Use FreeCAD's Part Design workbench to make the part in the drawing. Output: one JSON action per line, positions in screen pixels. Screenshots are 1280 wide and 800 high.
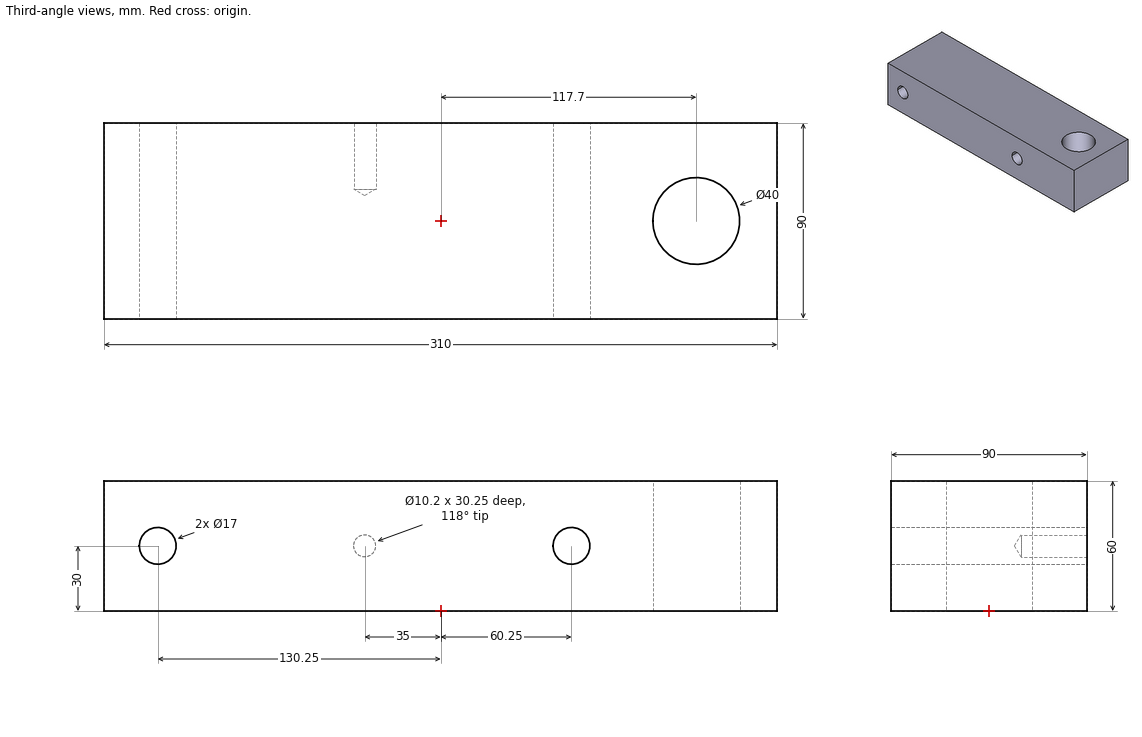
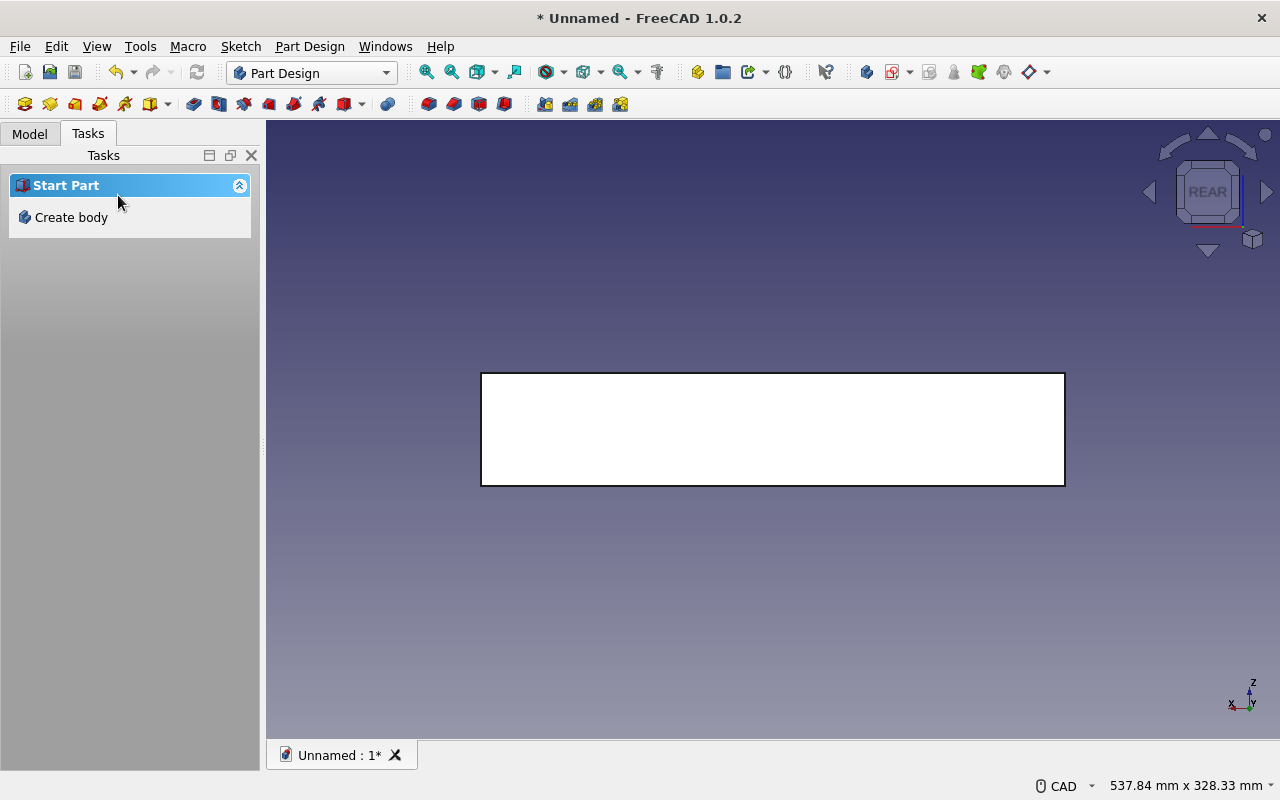
{"action": "left_click", "coordinate": [606, 429]}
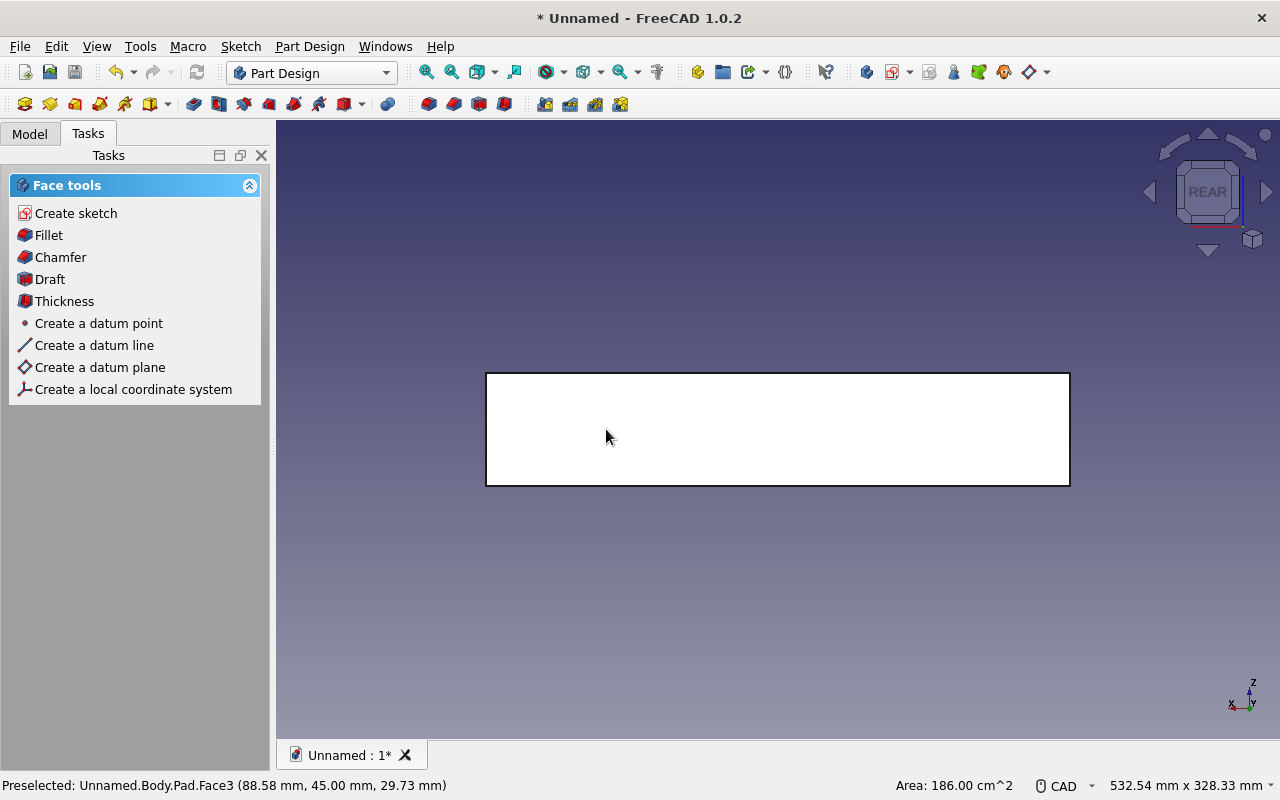
{"action": "left_click", "coordinate": [892, 72]}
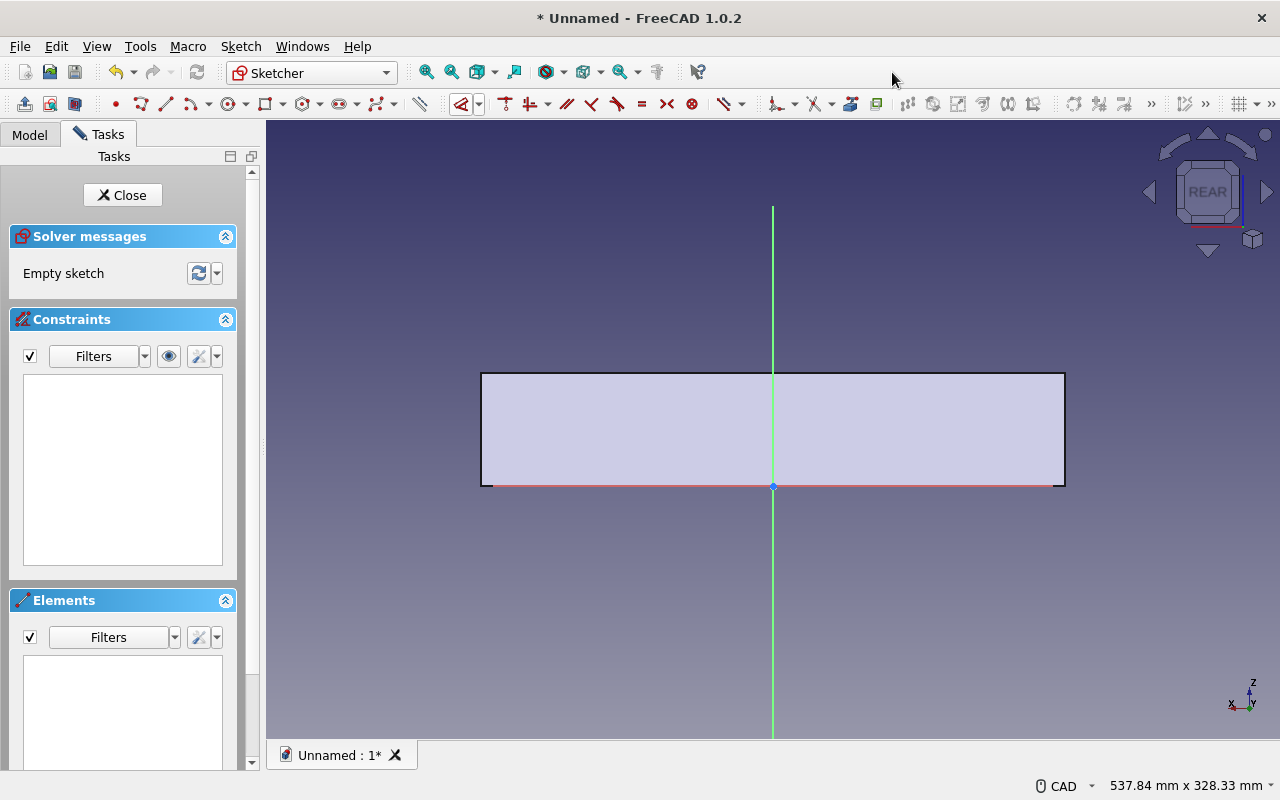
{"action": "scroll", "coordinate": [1112, 491], "scroll_direction": "up", "scroll_amount": 2}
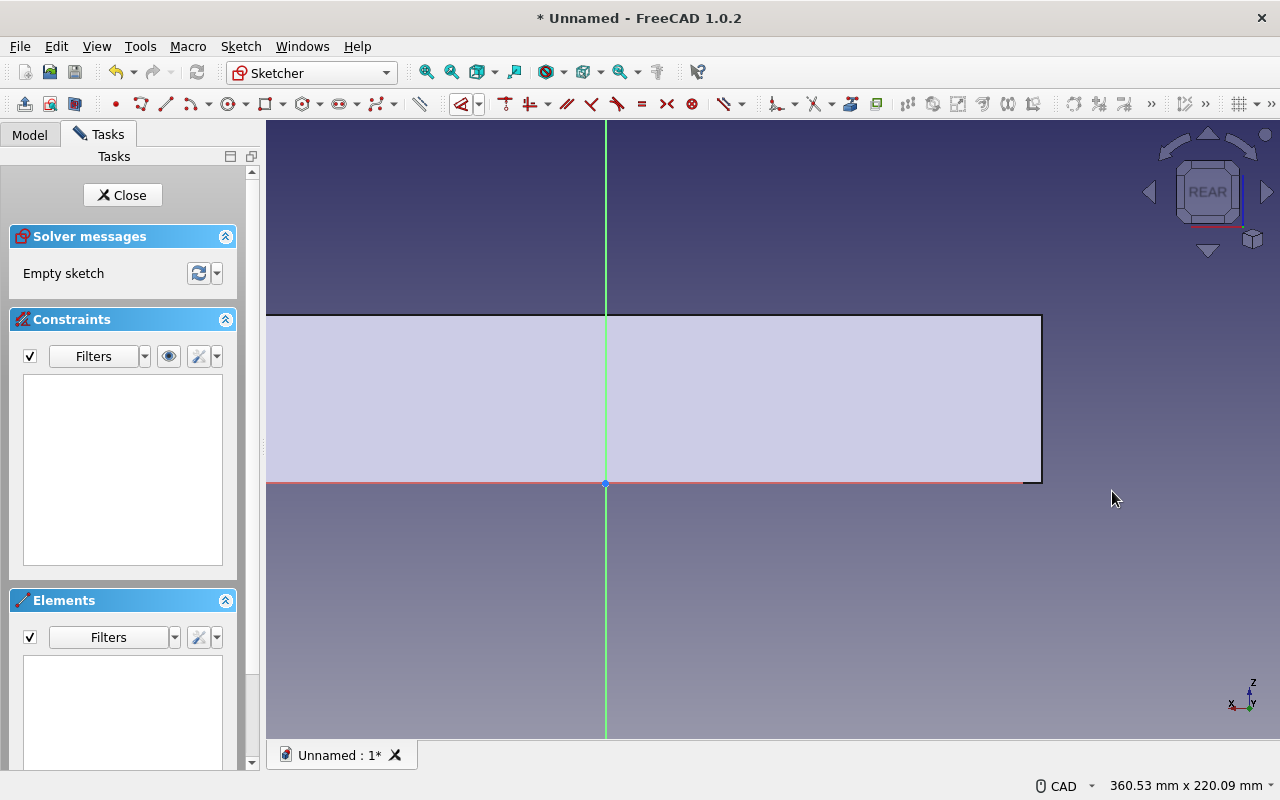
{"action": "key", "text": "g c"}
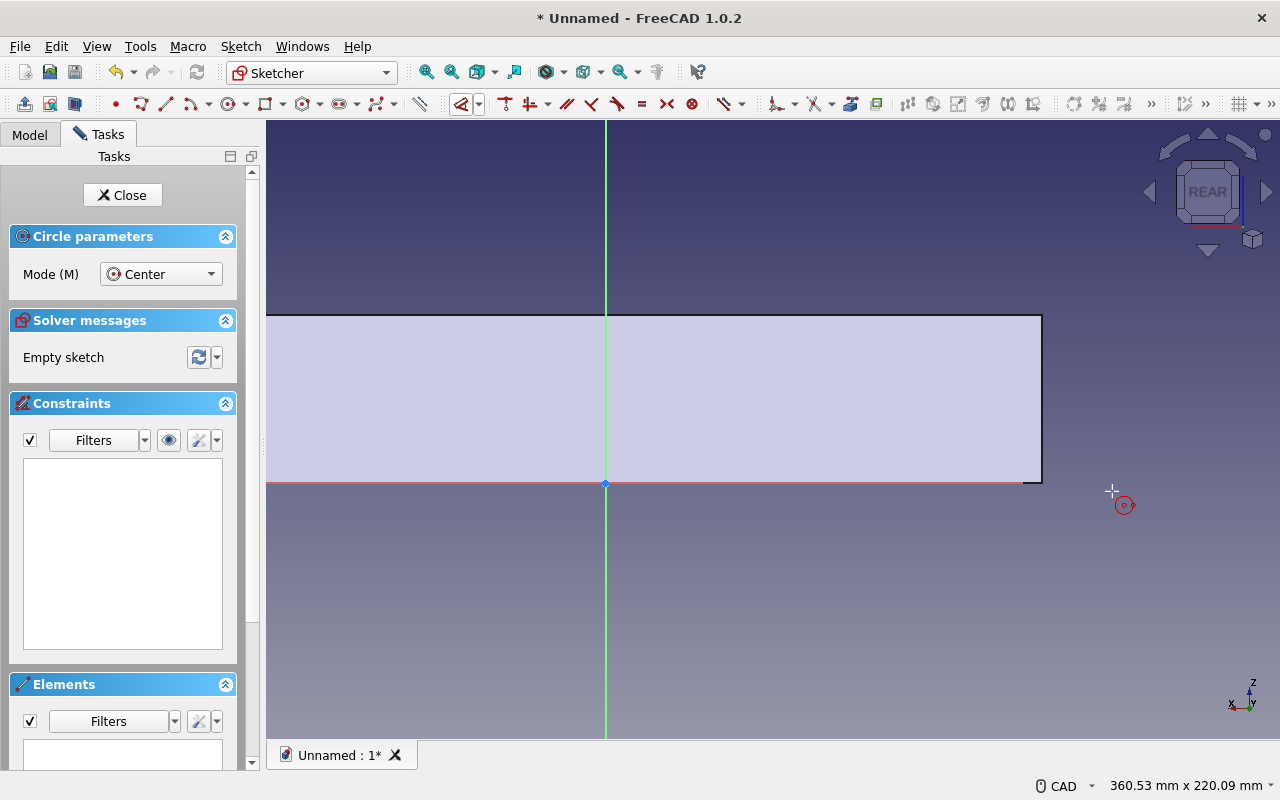
{"action": "left_click", "coordinate": [972, 399]}
{"action": "left_click", "coordinate": [989, 382]}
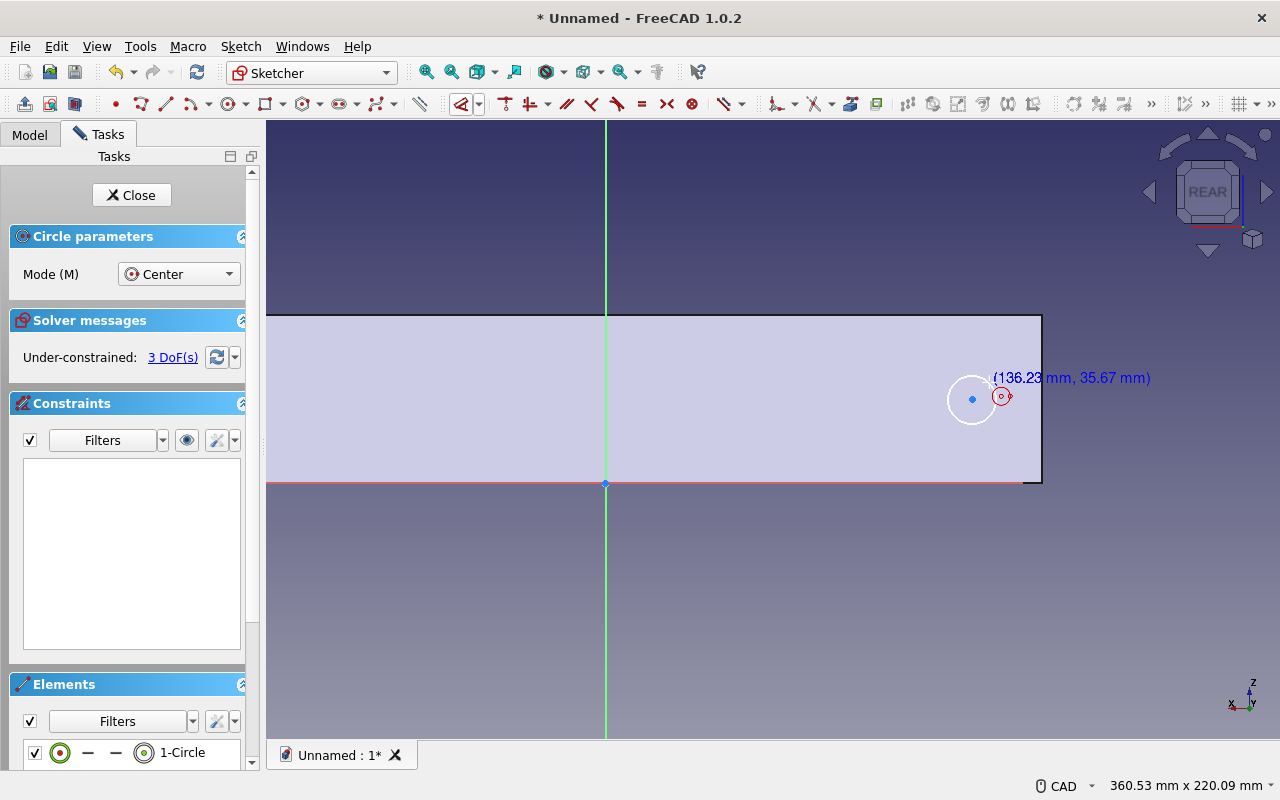
{"action": "left_click", "coordinate": [436, 399]}
{"action": "left_click", "coordinate": [453, 382]}
{"action": "key", "text": "Escape"}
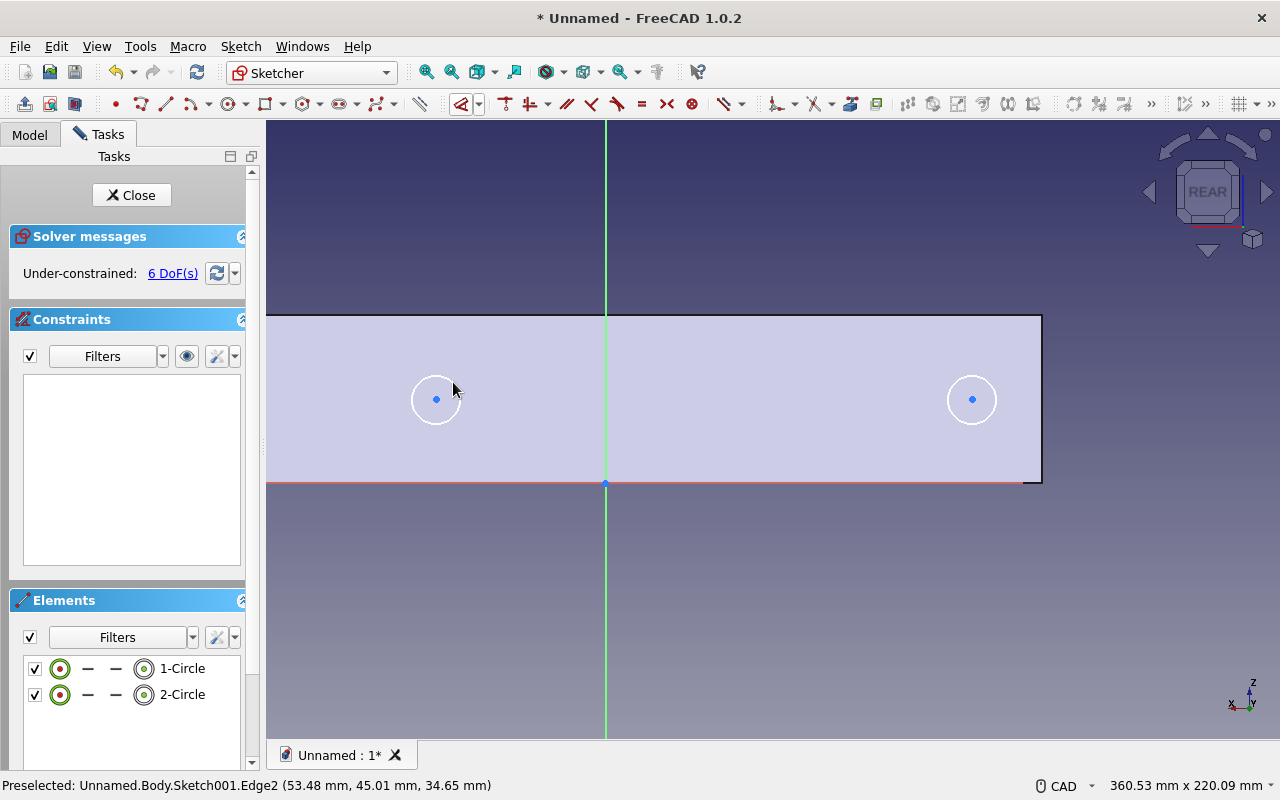
{"action": "left_click", "coordinate": [989, 383]}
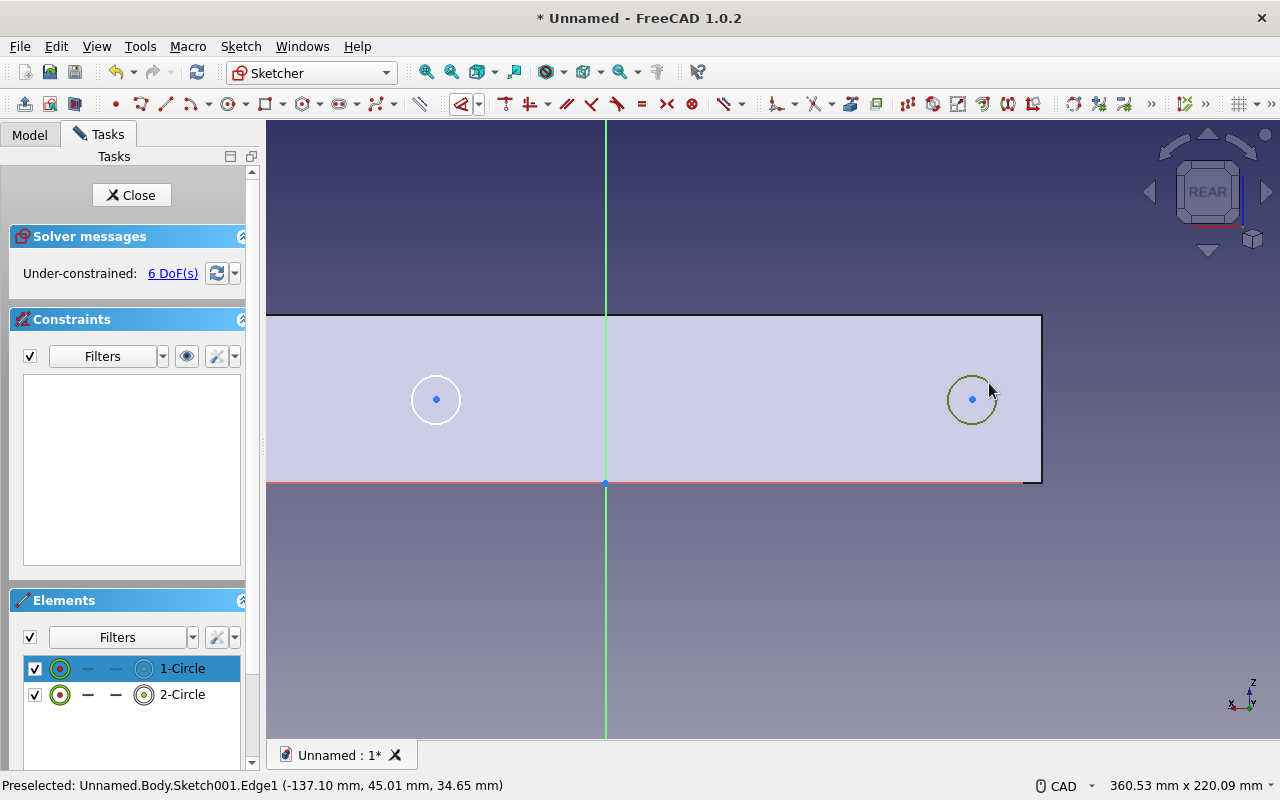
{"action": "left_click", "coordinate": [453, 383]}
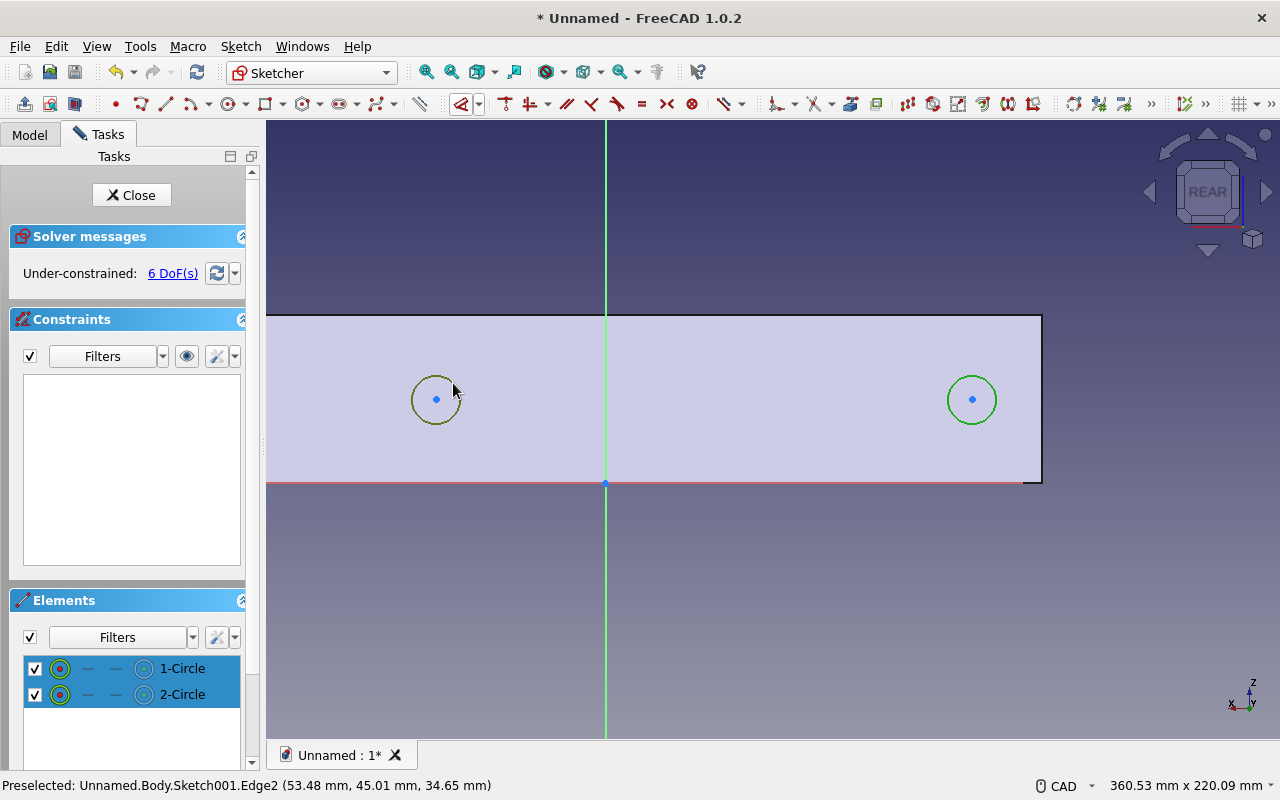
{"action": "key", "text": "e"}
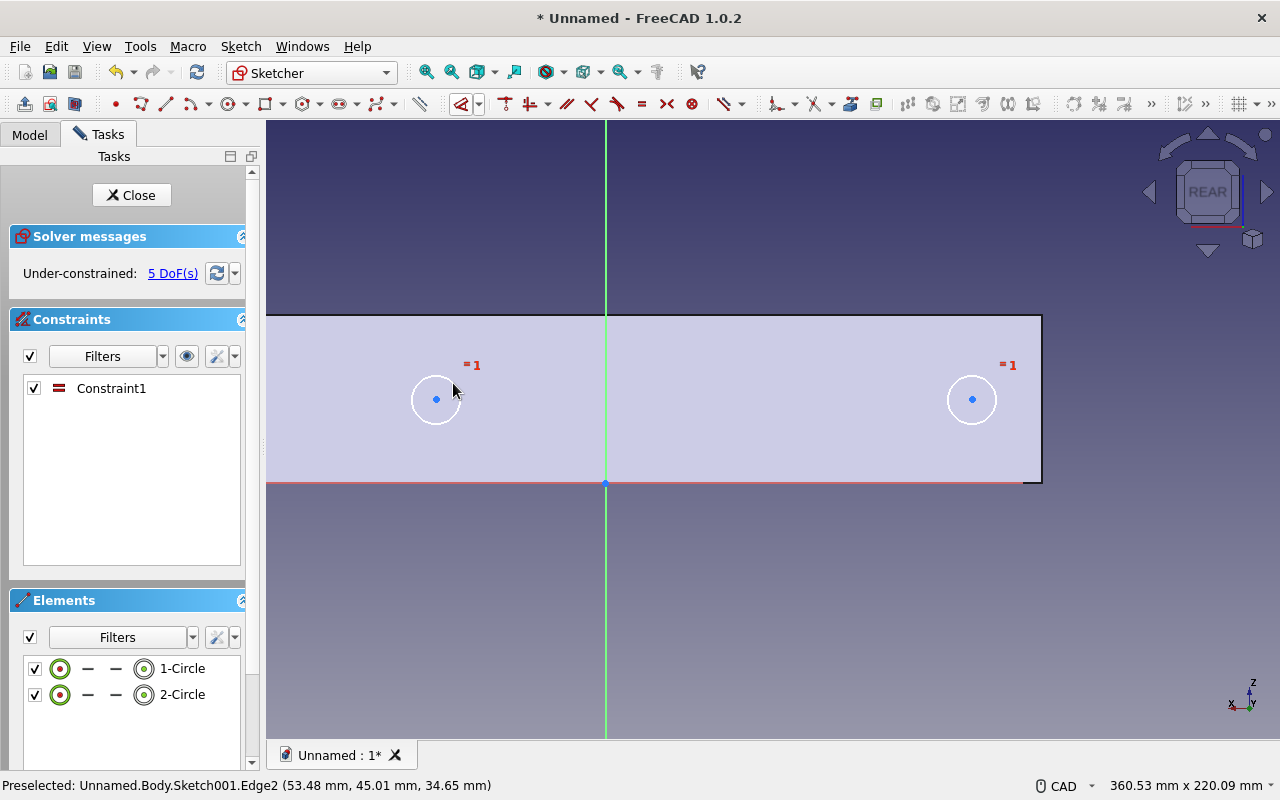
{"action": "left_click", "coordinate": [972, 400]}